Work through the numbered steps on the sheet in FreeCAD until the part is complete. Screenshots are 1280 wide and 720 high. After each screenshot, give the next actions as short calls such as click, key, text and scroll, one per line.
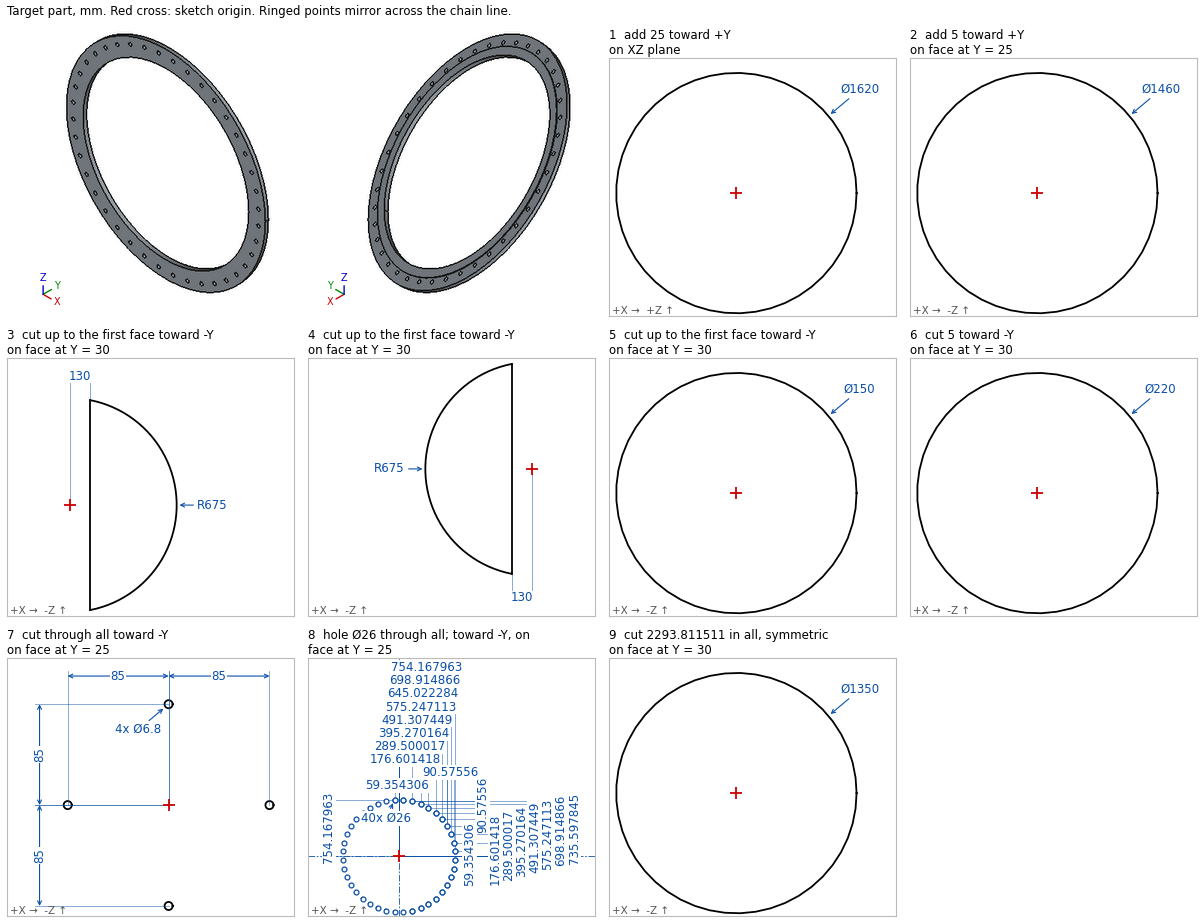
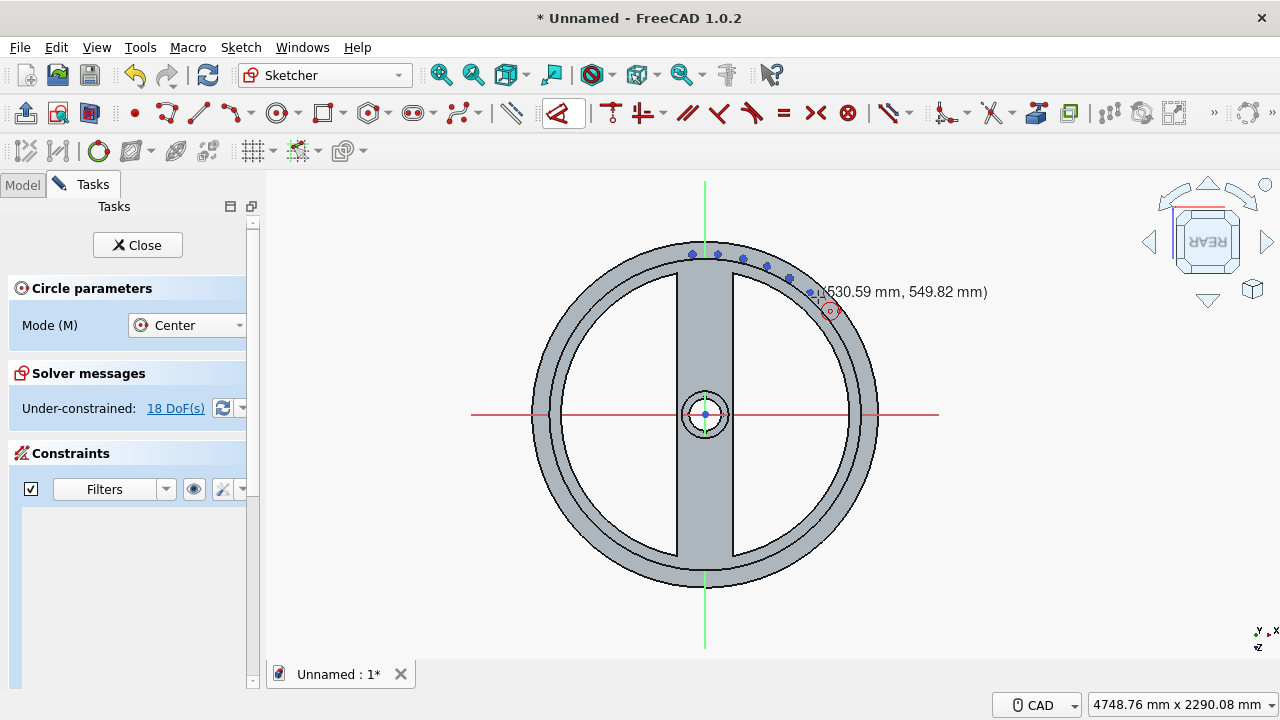
click(828, 310)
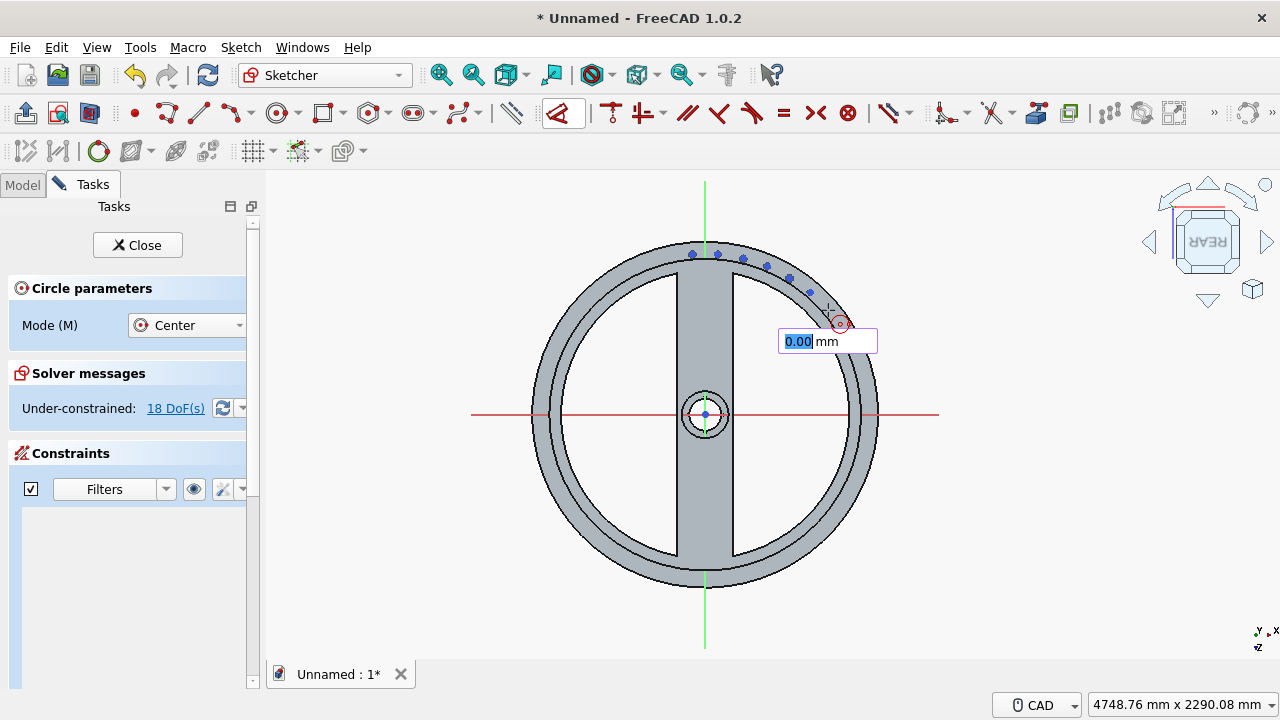
scroll(830, 308, up, 9)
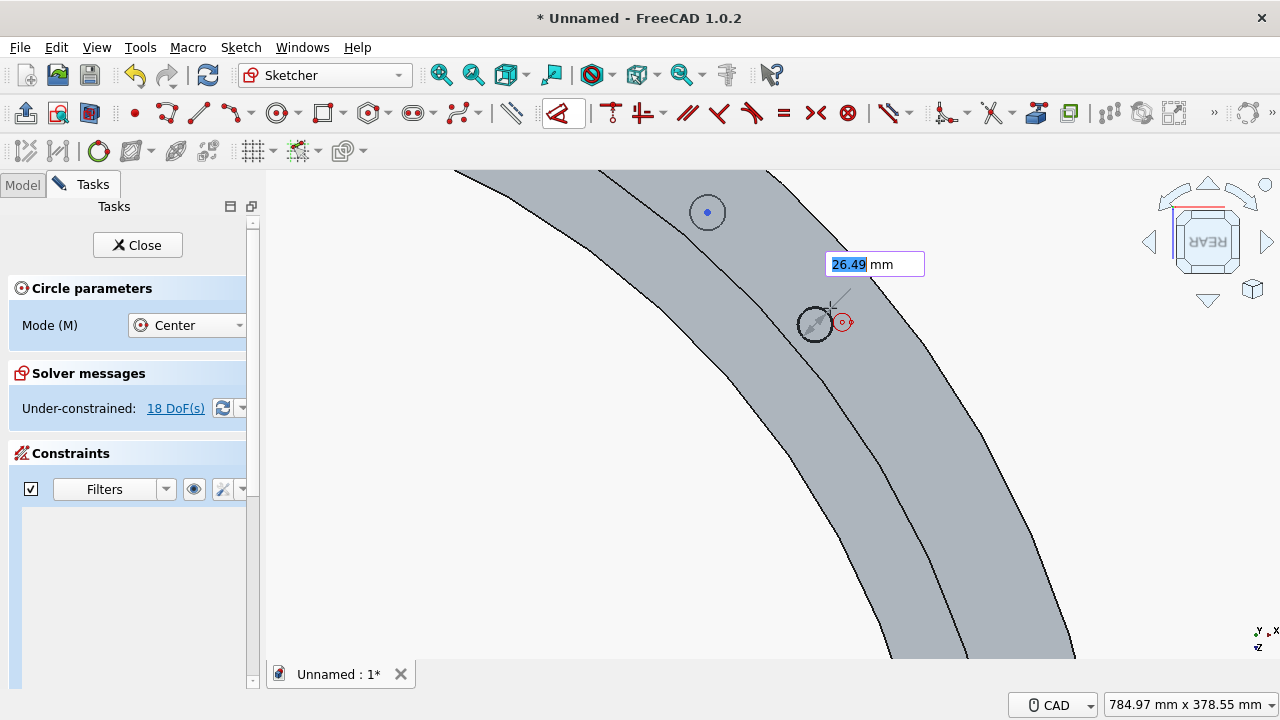
click(827, 306)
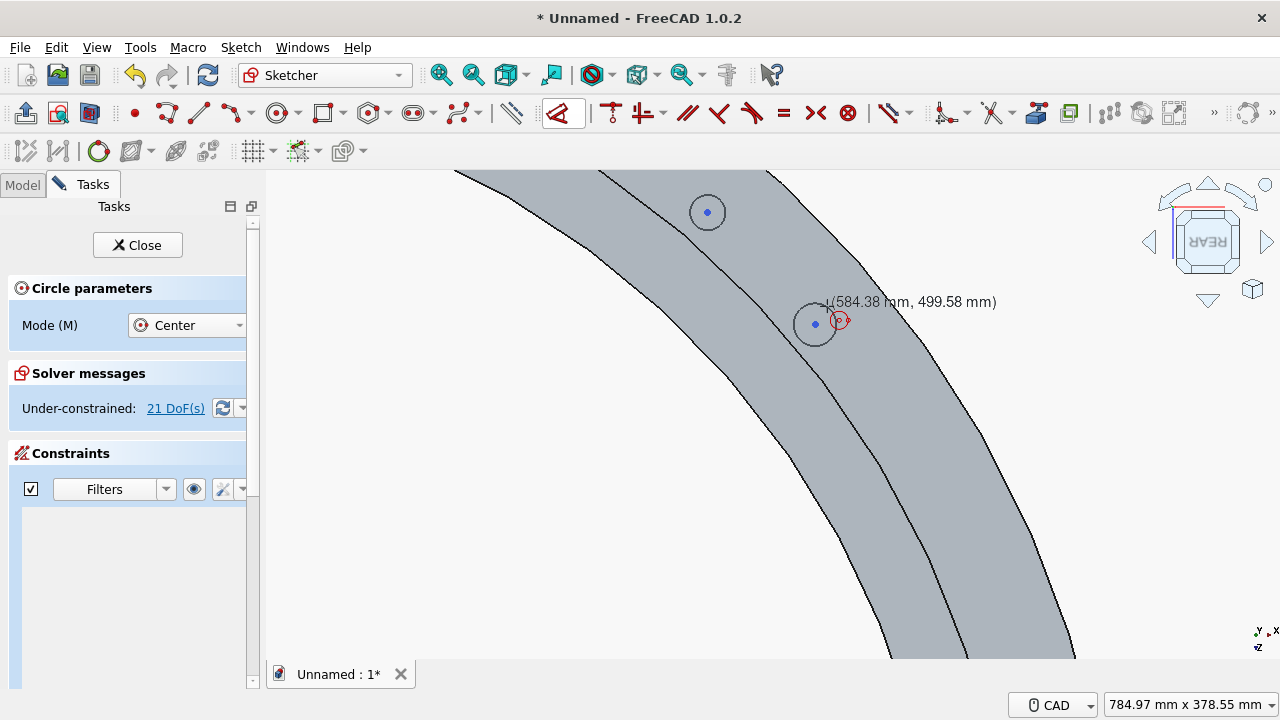
scroll(905, 442, up, 2)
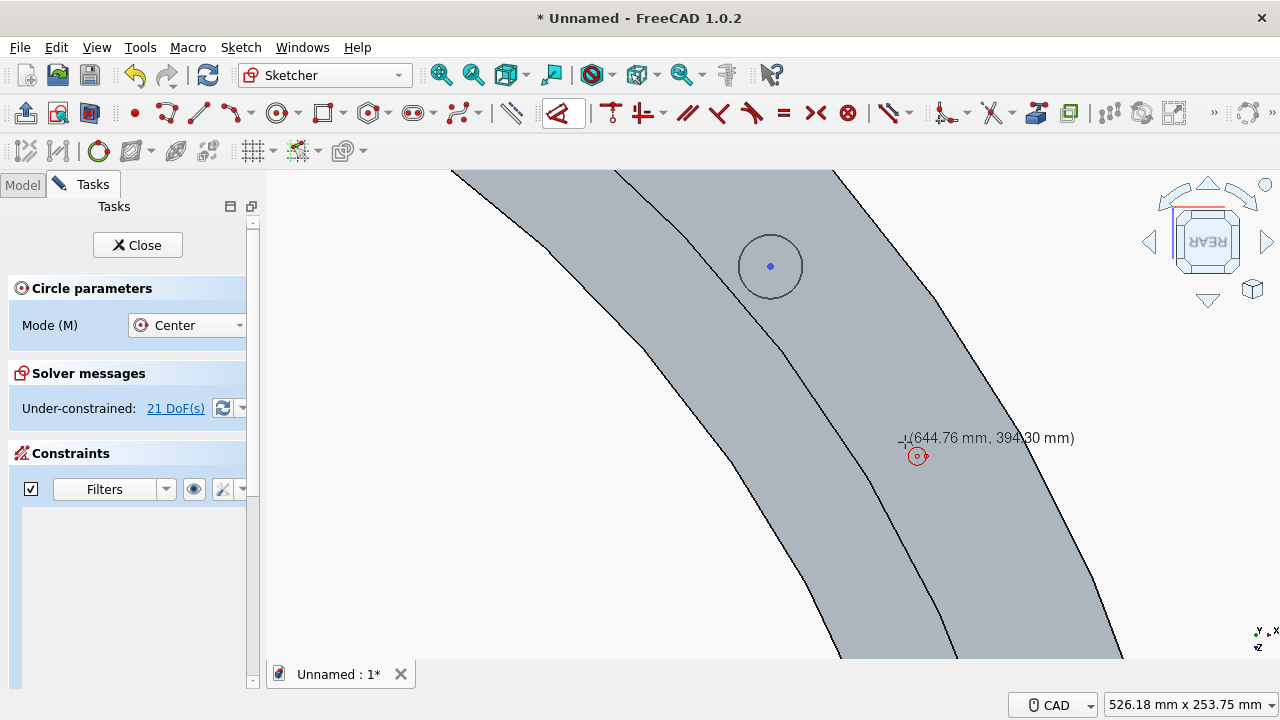
scroll(834, 316, down, 11)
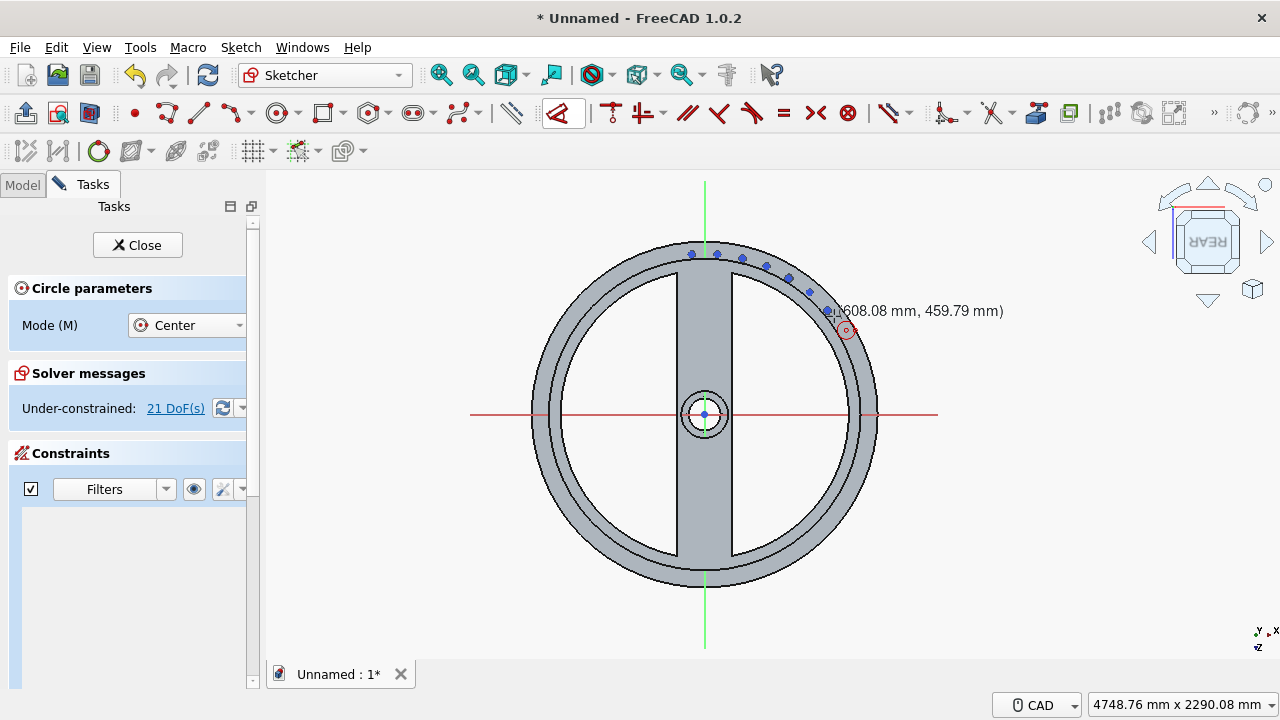
click(842, 330)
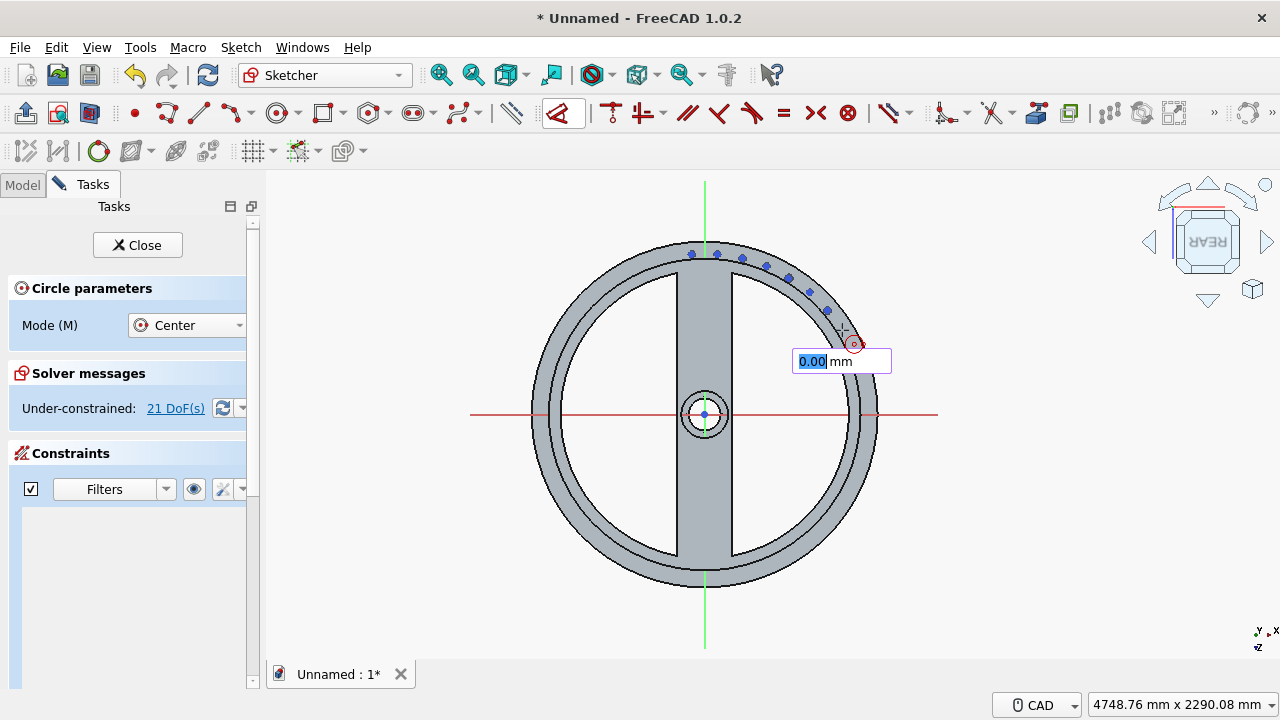
scroll(844, 328, up, 9)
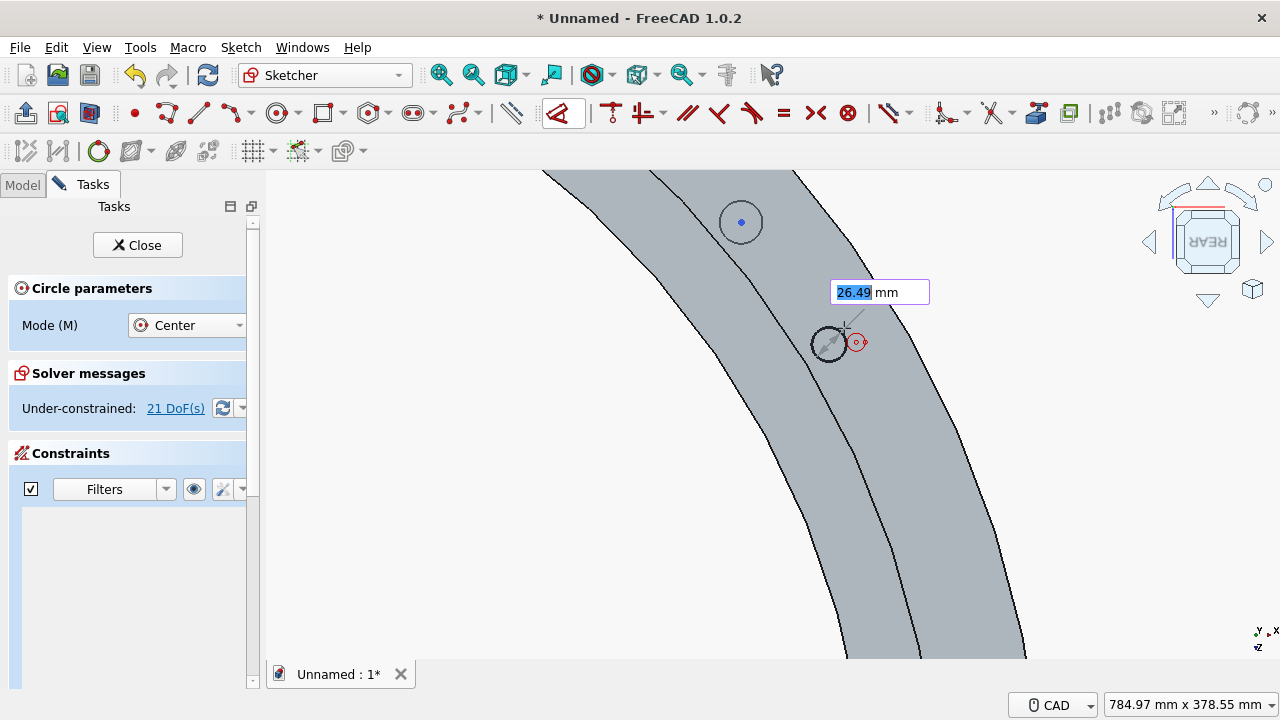
click(843, 328)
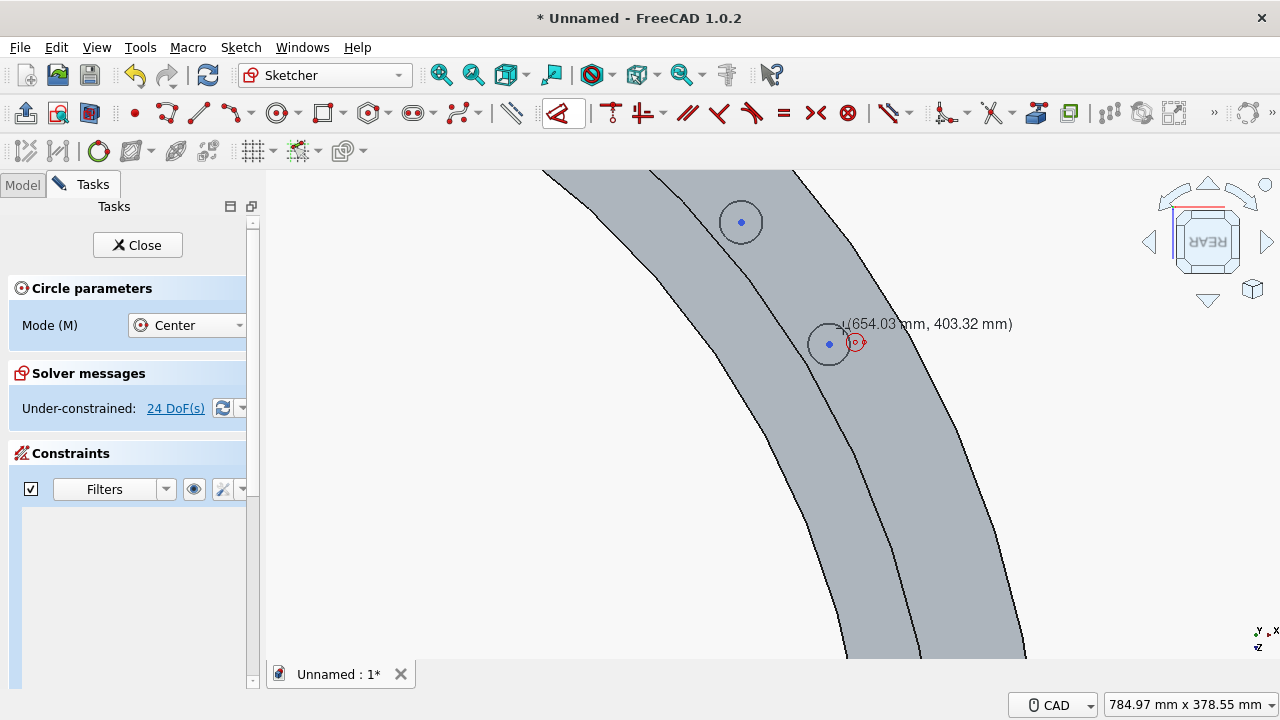
scroll(901, 476, up, 2)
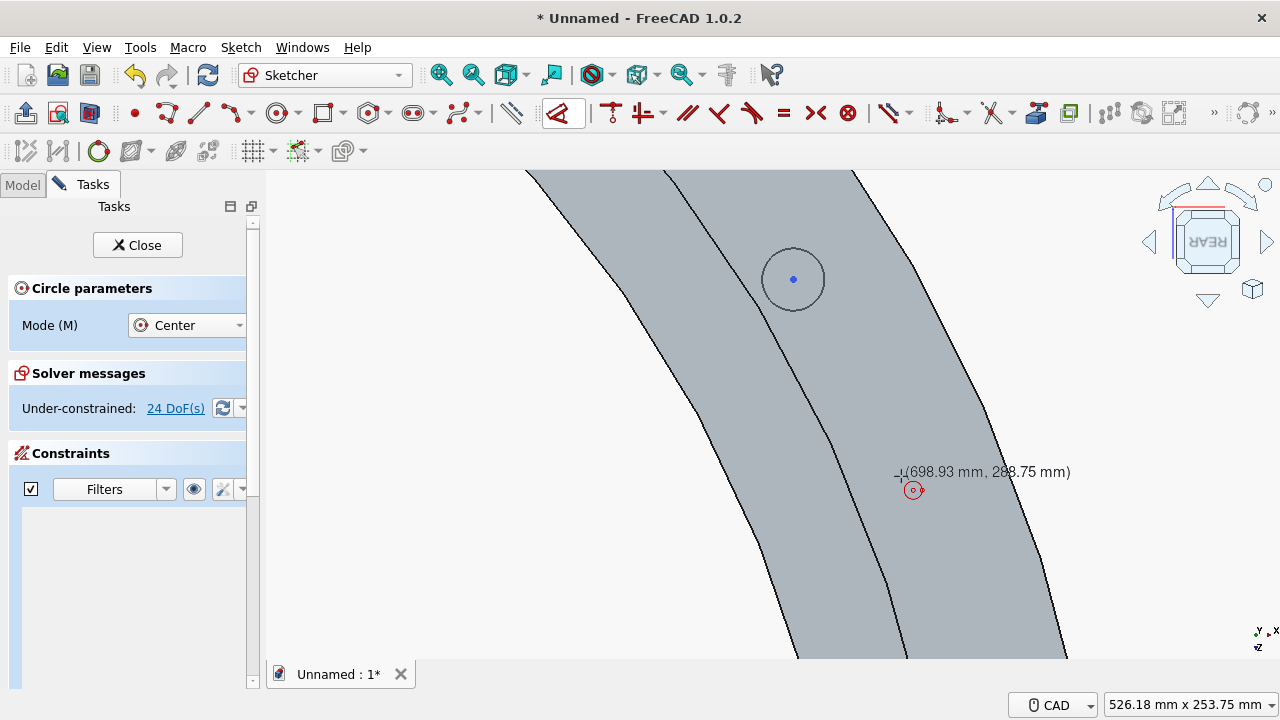
scroll(848, 337, down, 11)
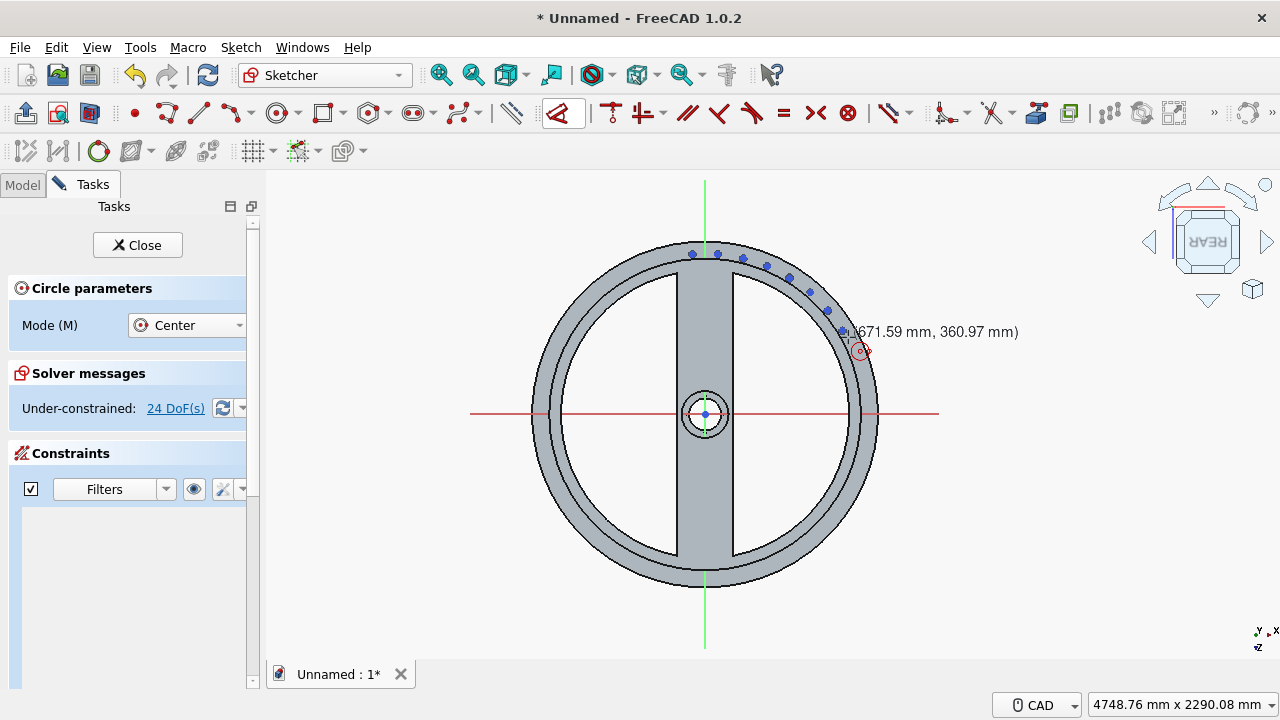
click(854, 353)